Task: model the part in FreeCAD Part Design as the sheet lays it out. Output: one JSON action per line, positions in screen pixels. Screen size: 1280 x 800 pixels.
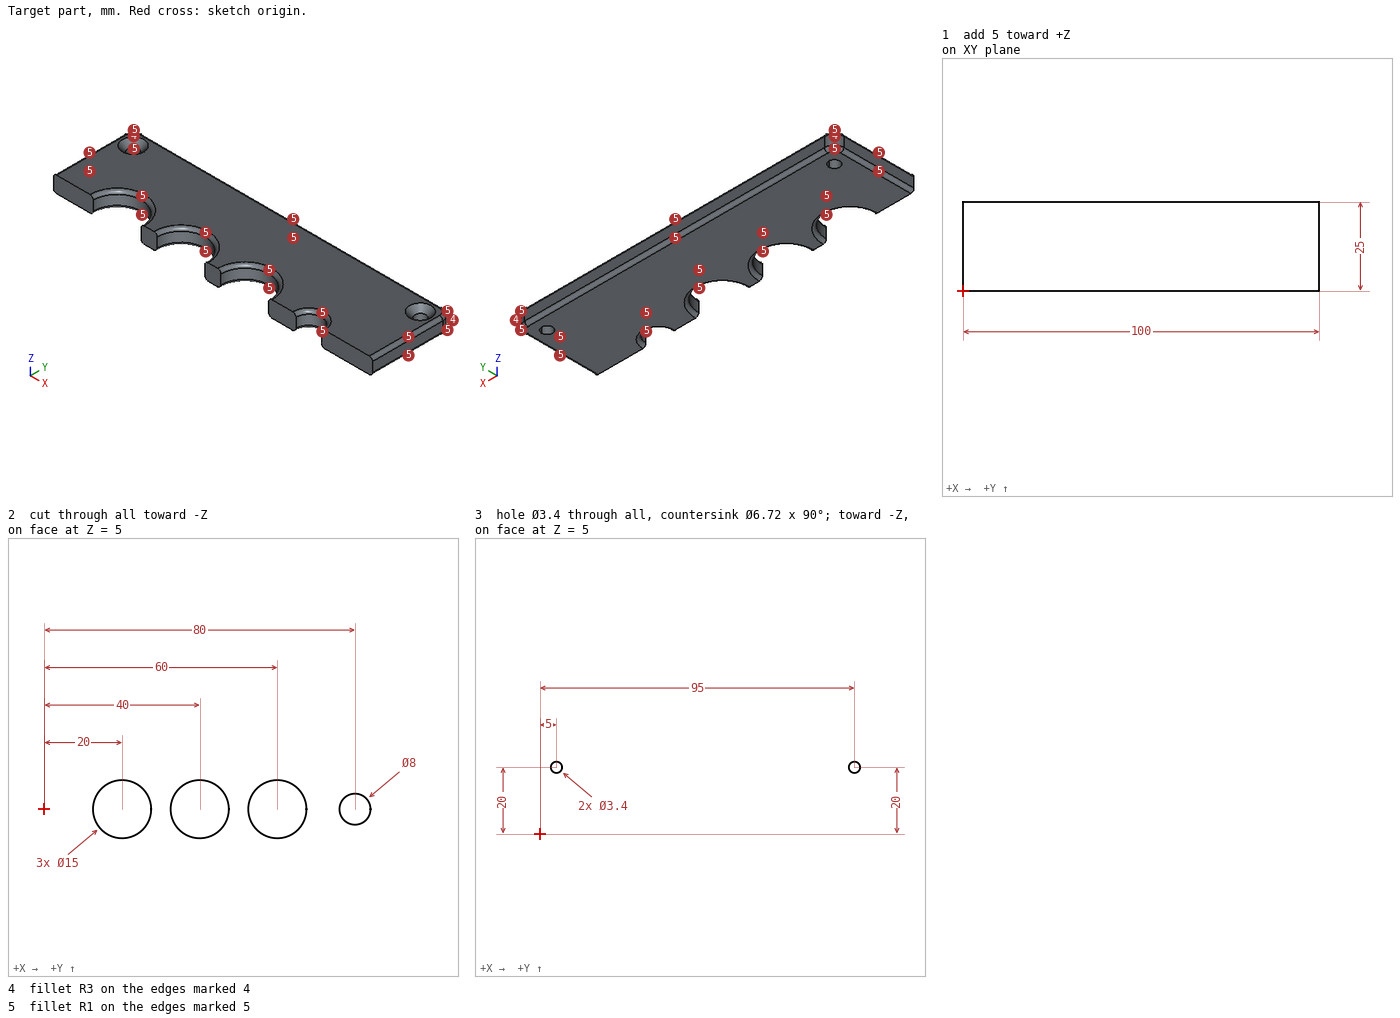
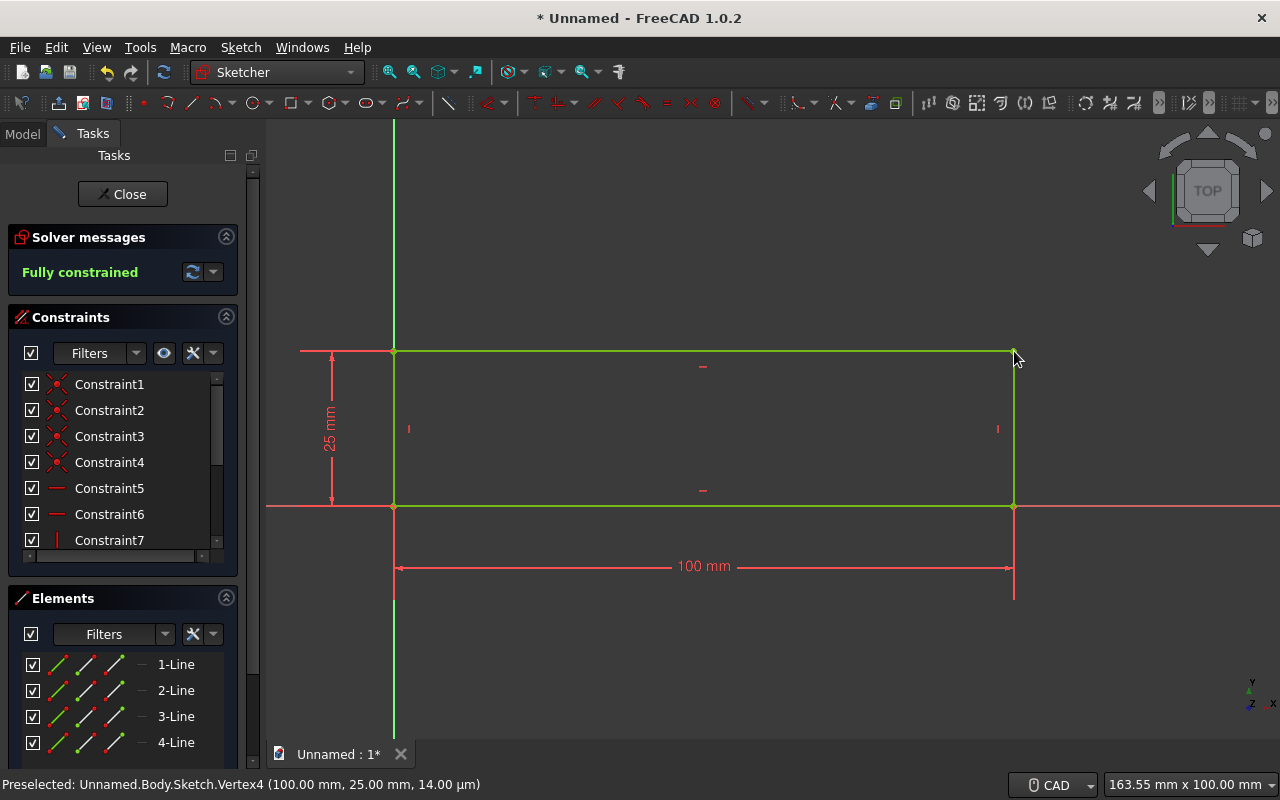
{"action": "left_click", "coordinate": [123, 194]}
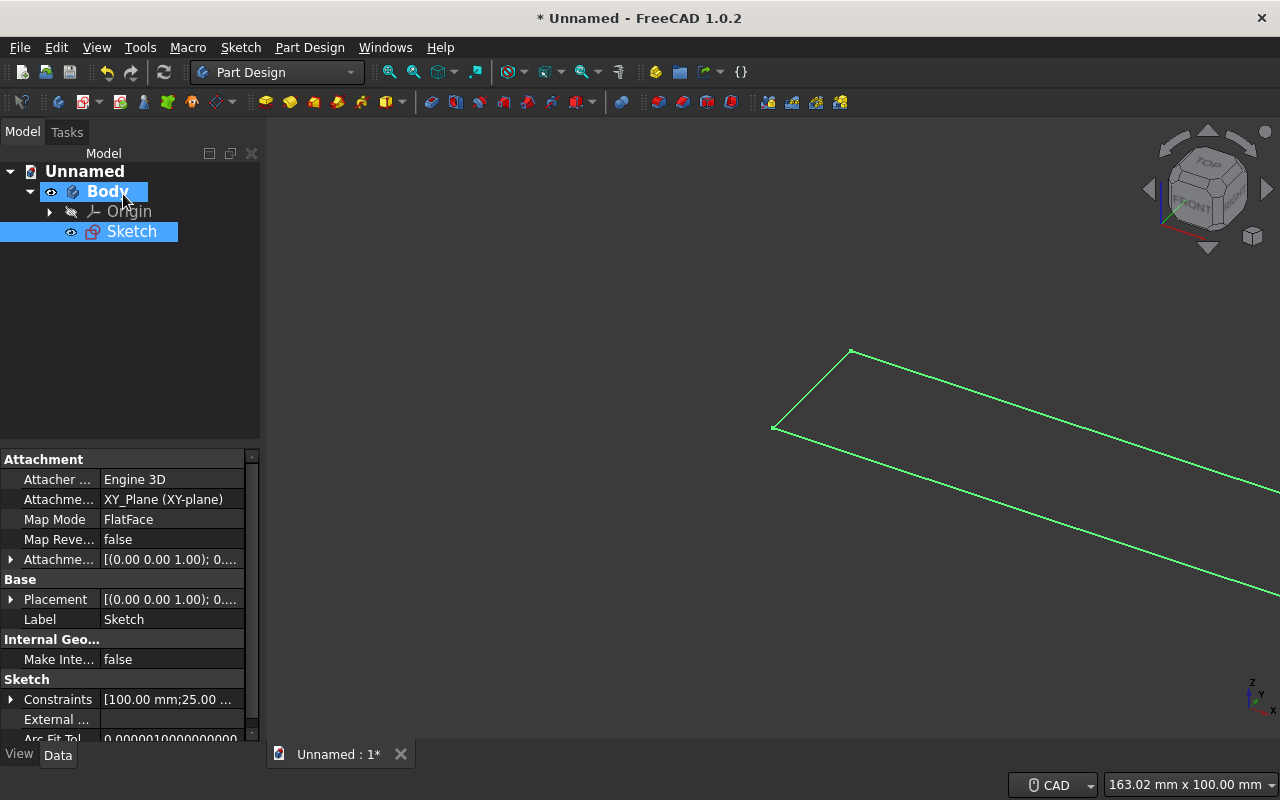
{"action": "left_click", "coordinate": [266, 102]}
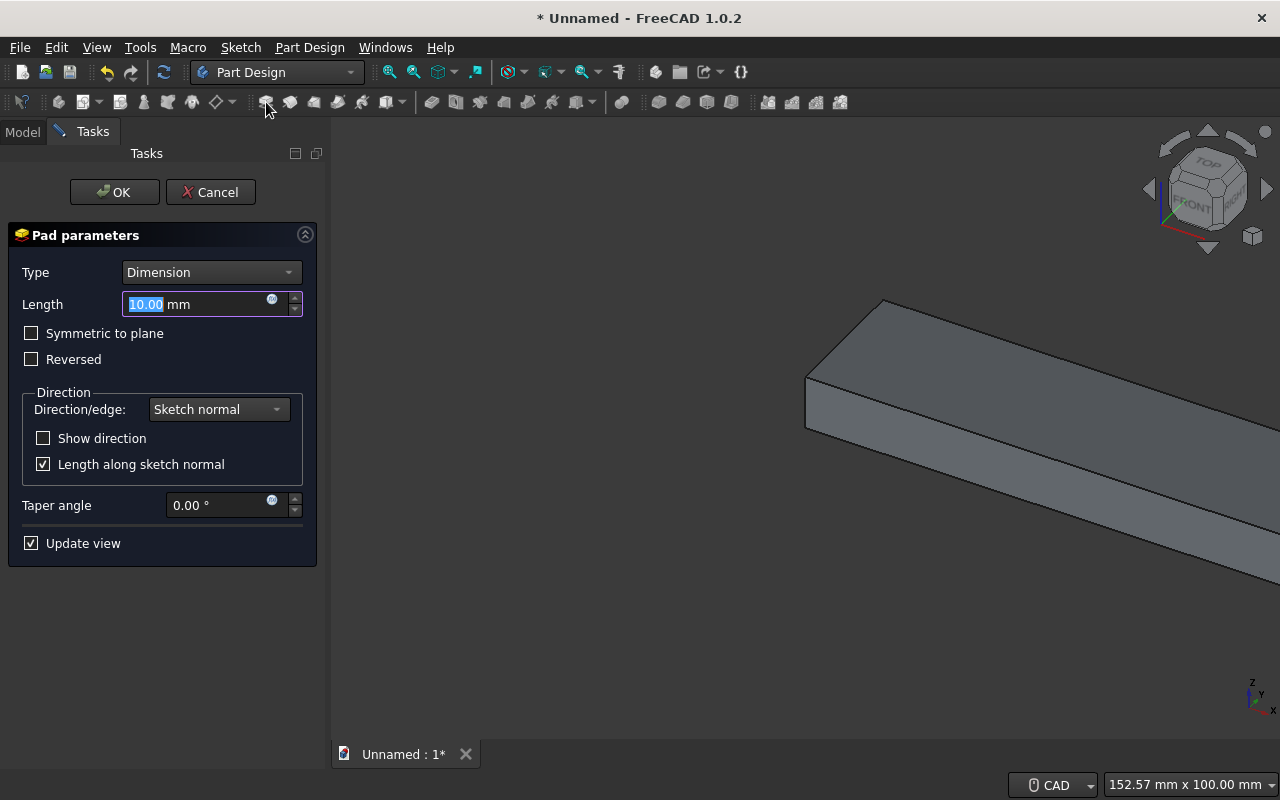
{"action": "type", "text": "5"}
{"action": "key", "text": "Tab"}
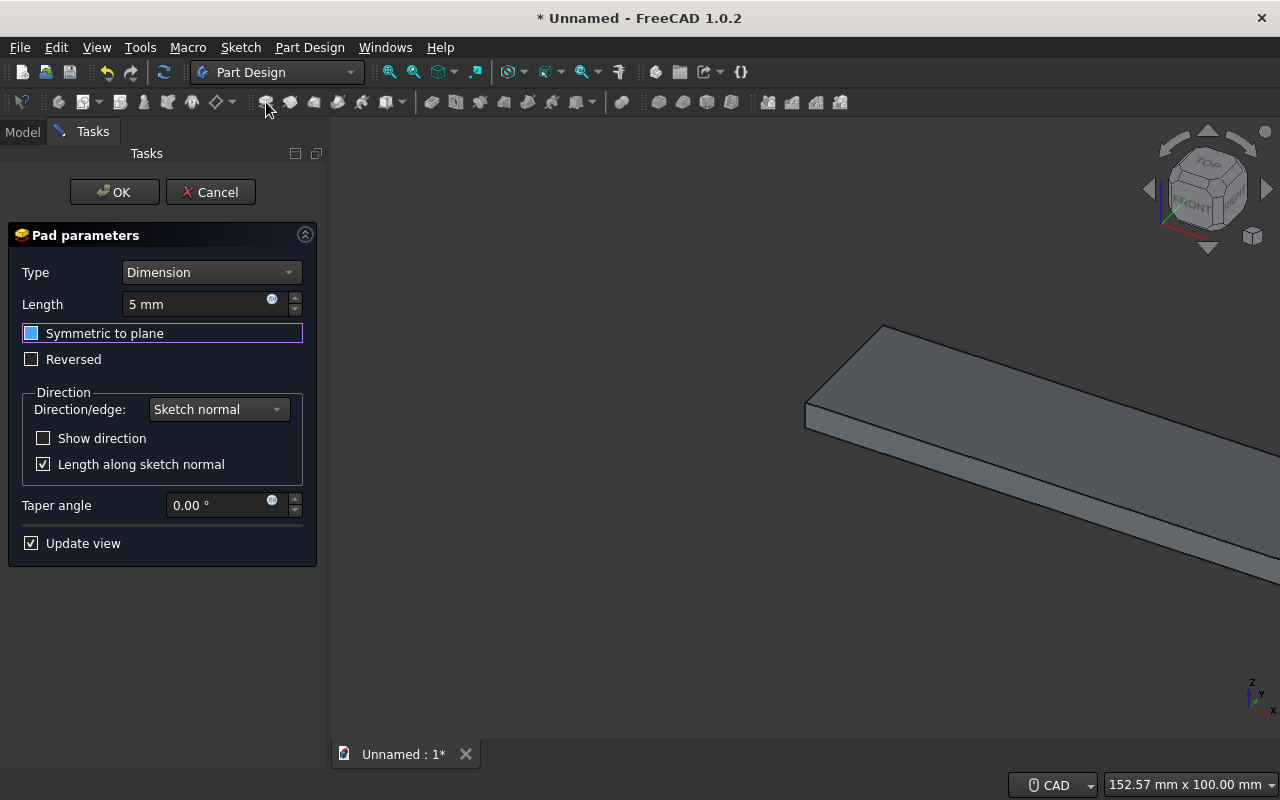
{"action": "left_click", "coordinate": [115, 192]}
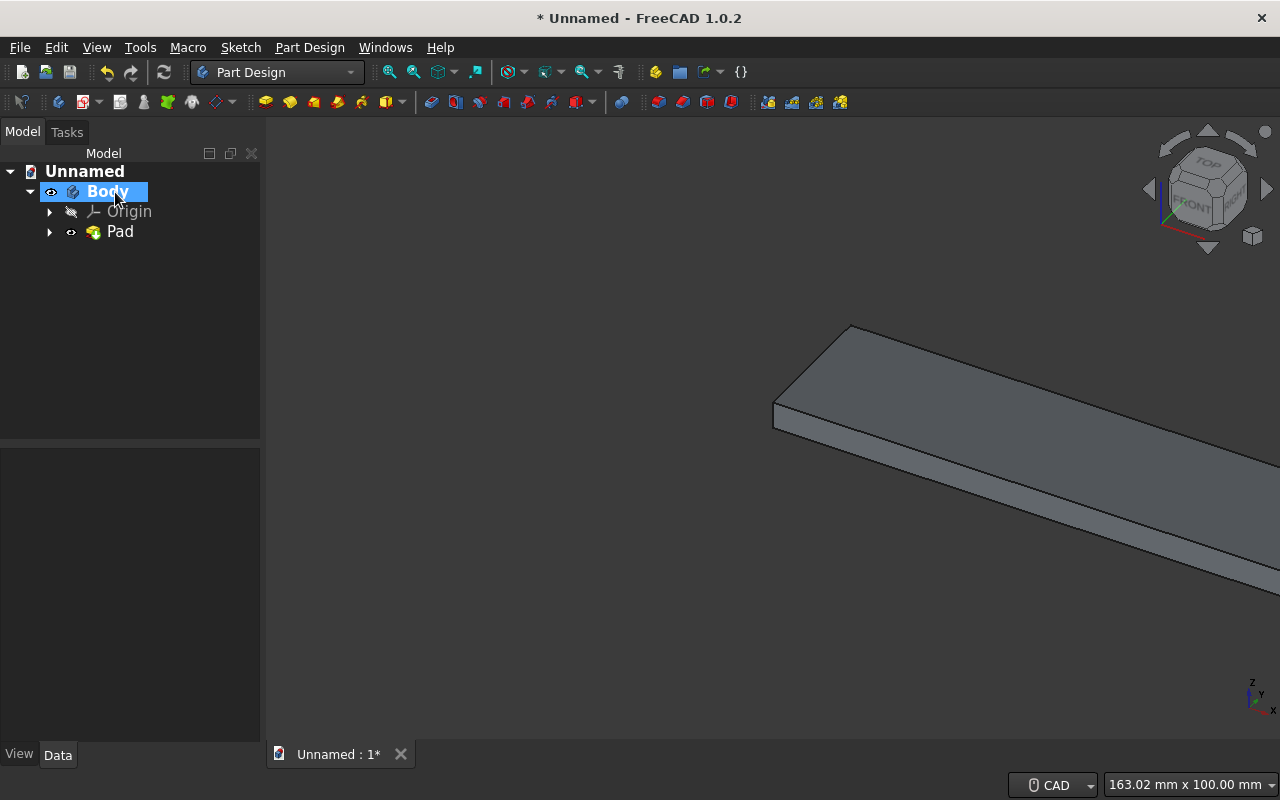
{"action": "left_click", "coordinate": [390, 72]}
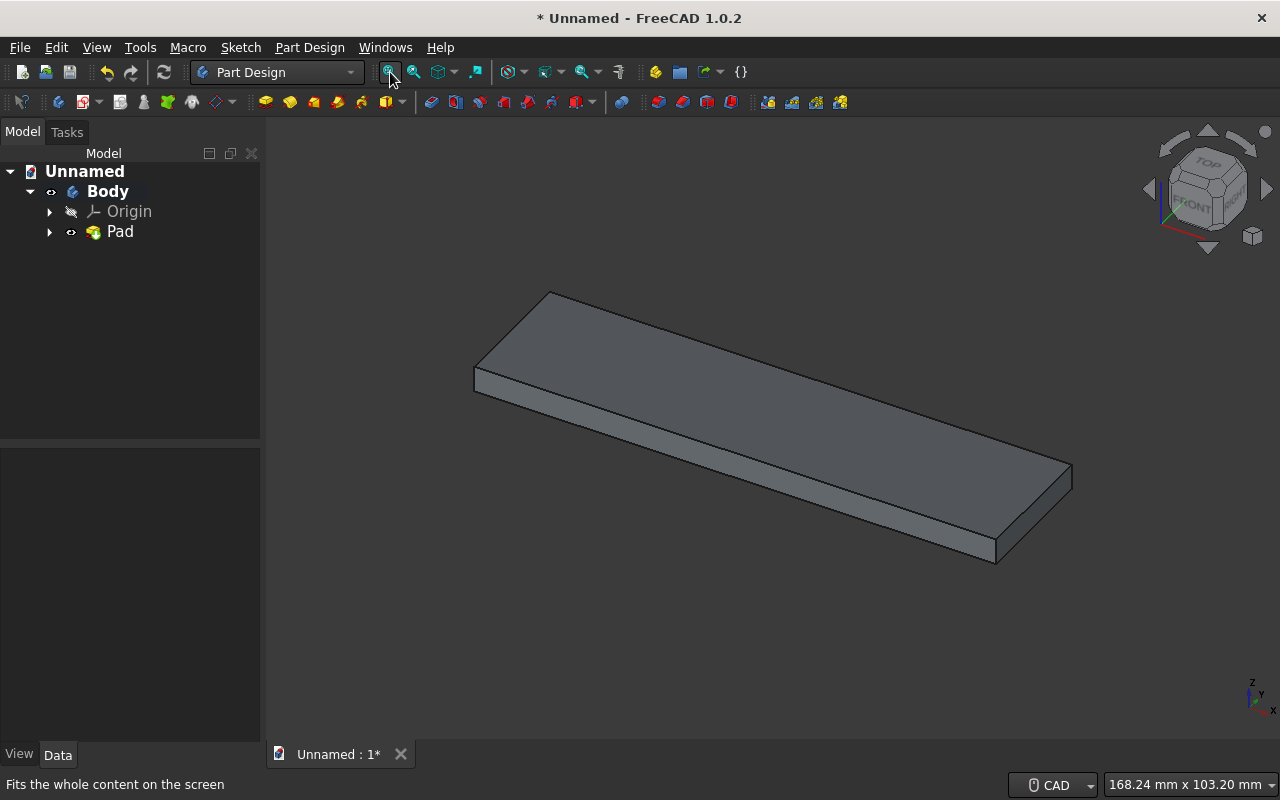
{"action": "left_click", "coordinate": [922, 464]}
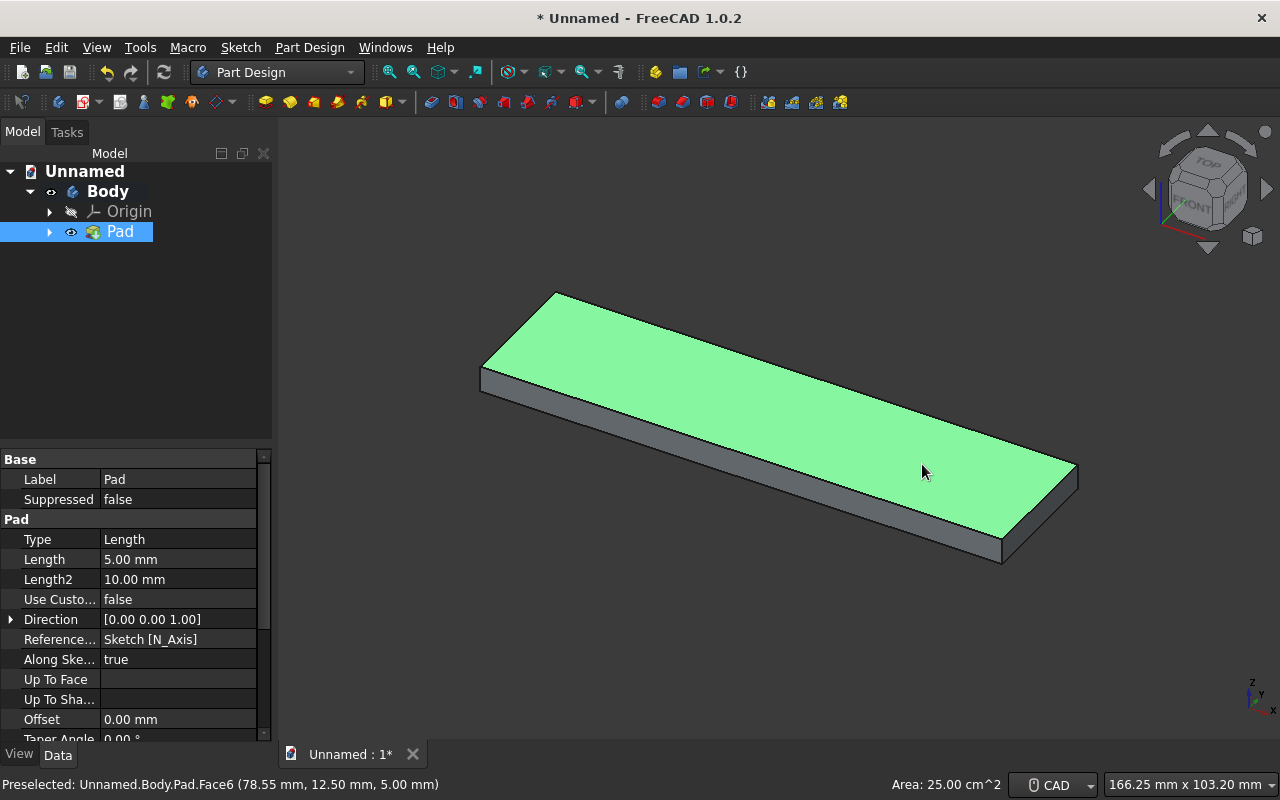
{"action": "left_click", "coordinate": [84, 102]}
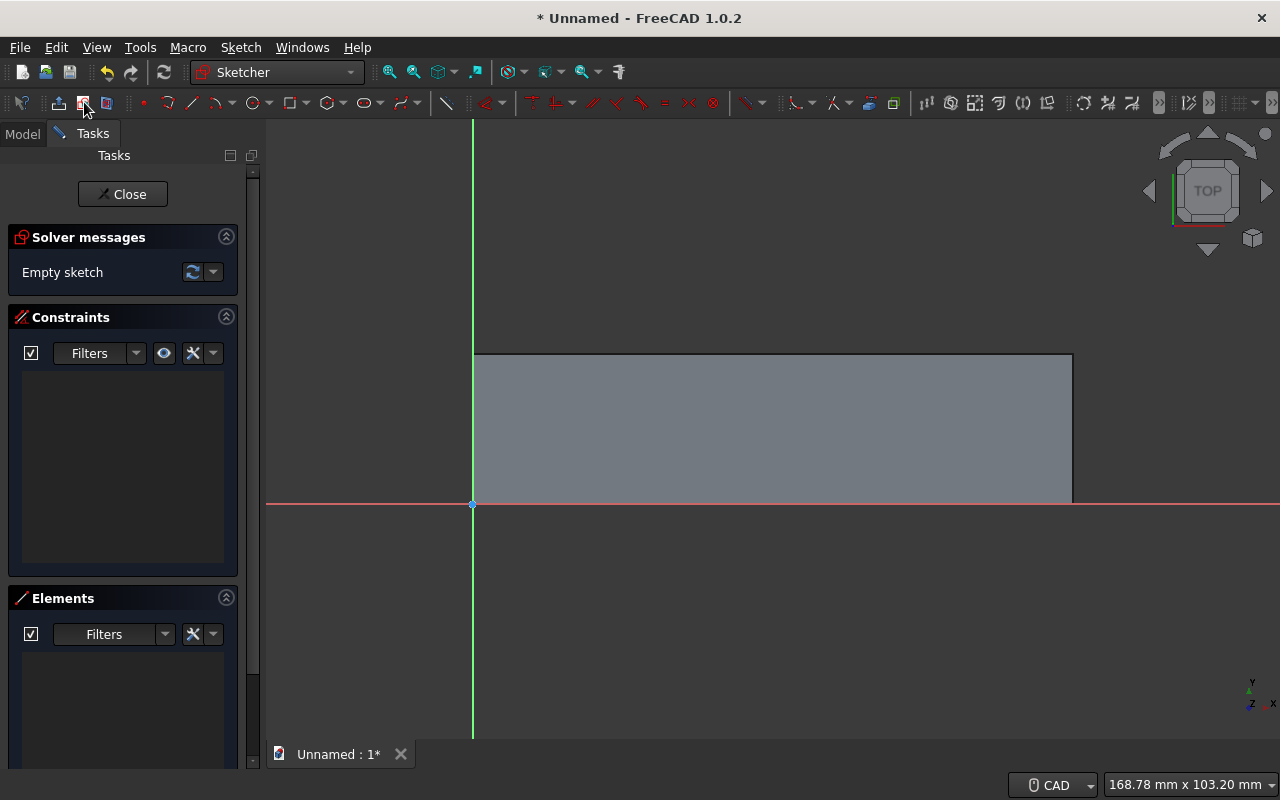
{"action": "left_click", "coordinate": [254, 104]}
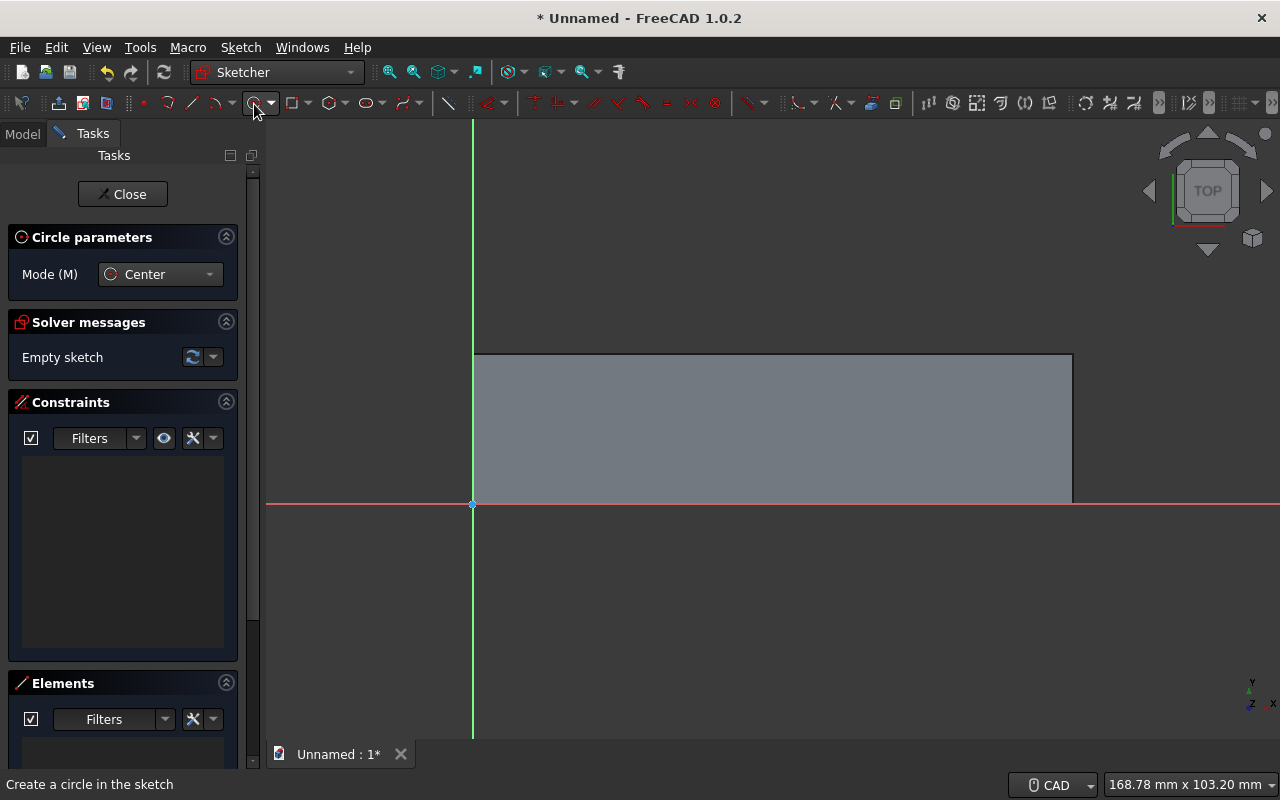
{"action": "left_click", "coordinate": [593, 504]}
{"action": "mouse_move", "coordinate": [625, 472]}